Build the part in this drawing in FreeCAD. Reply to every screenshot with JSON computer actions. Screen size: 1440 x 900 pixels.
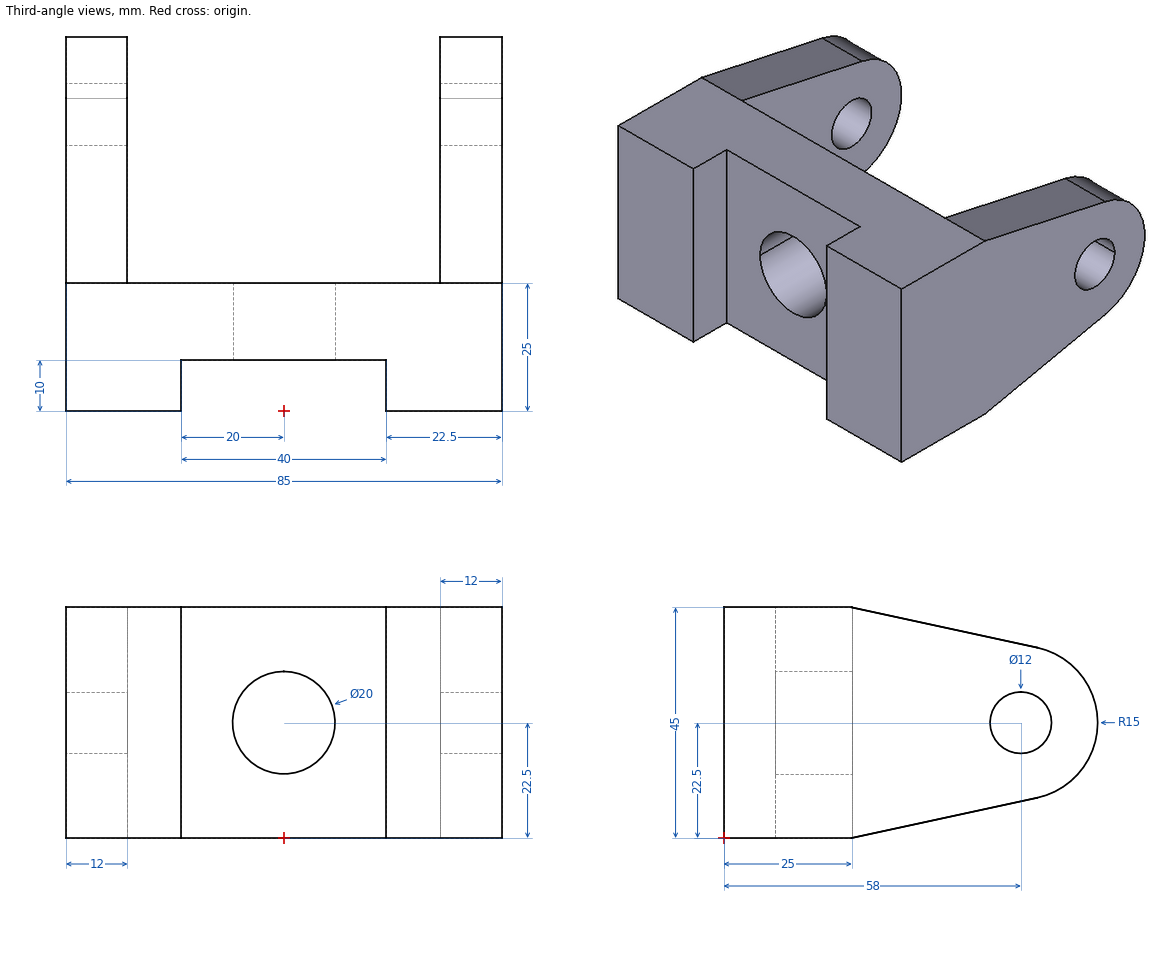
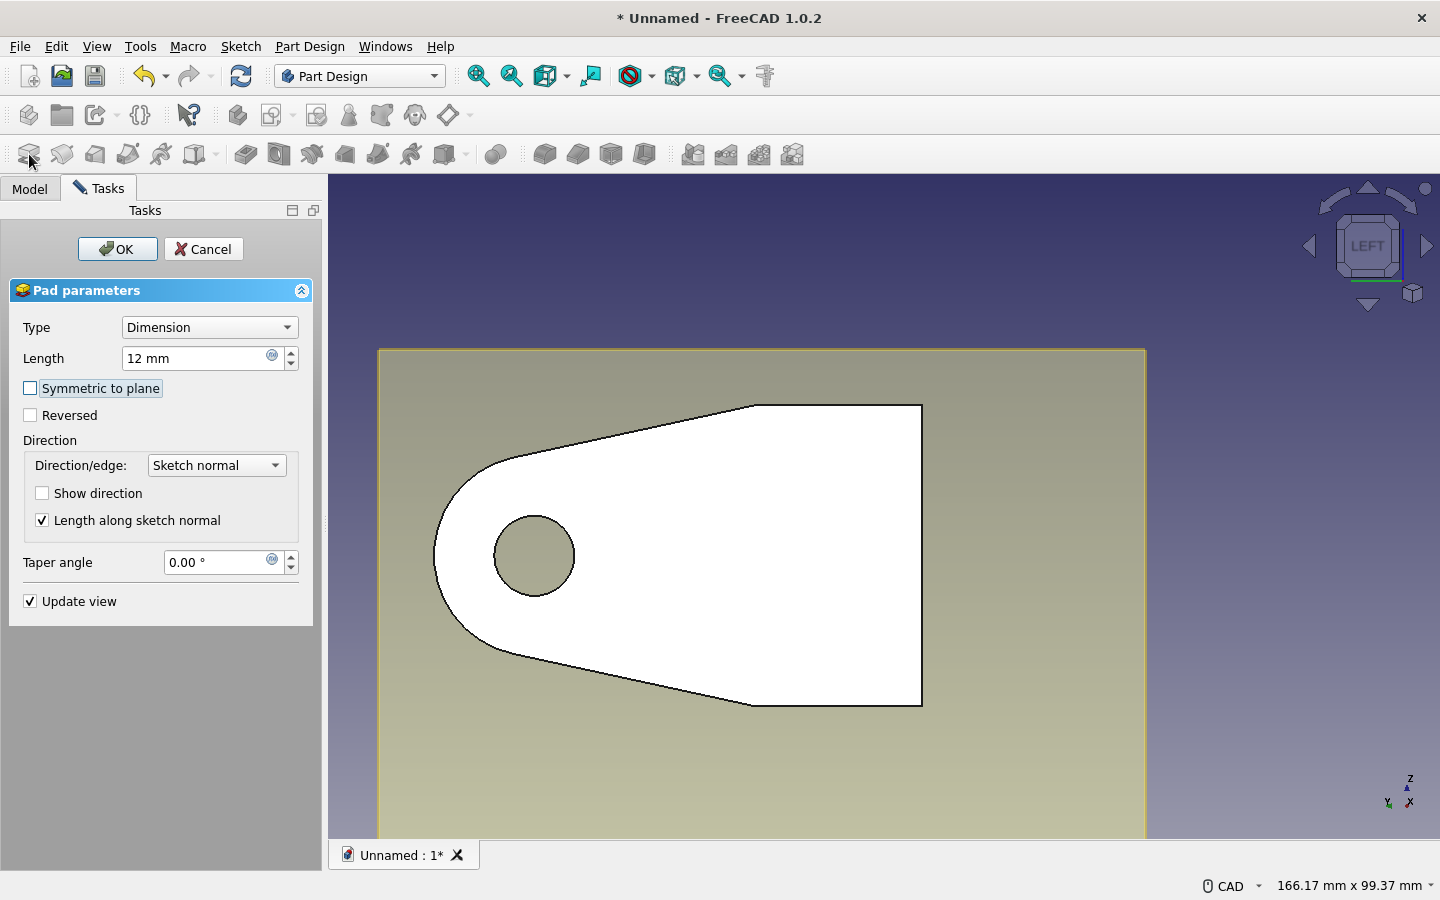
{"action": "left_click", "coordinate": [118, 249]}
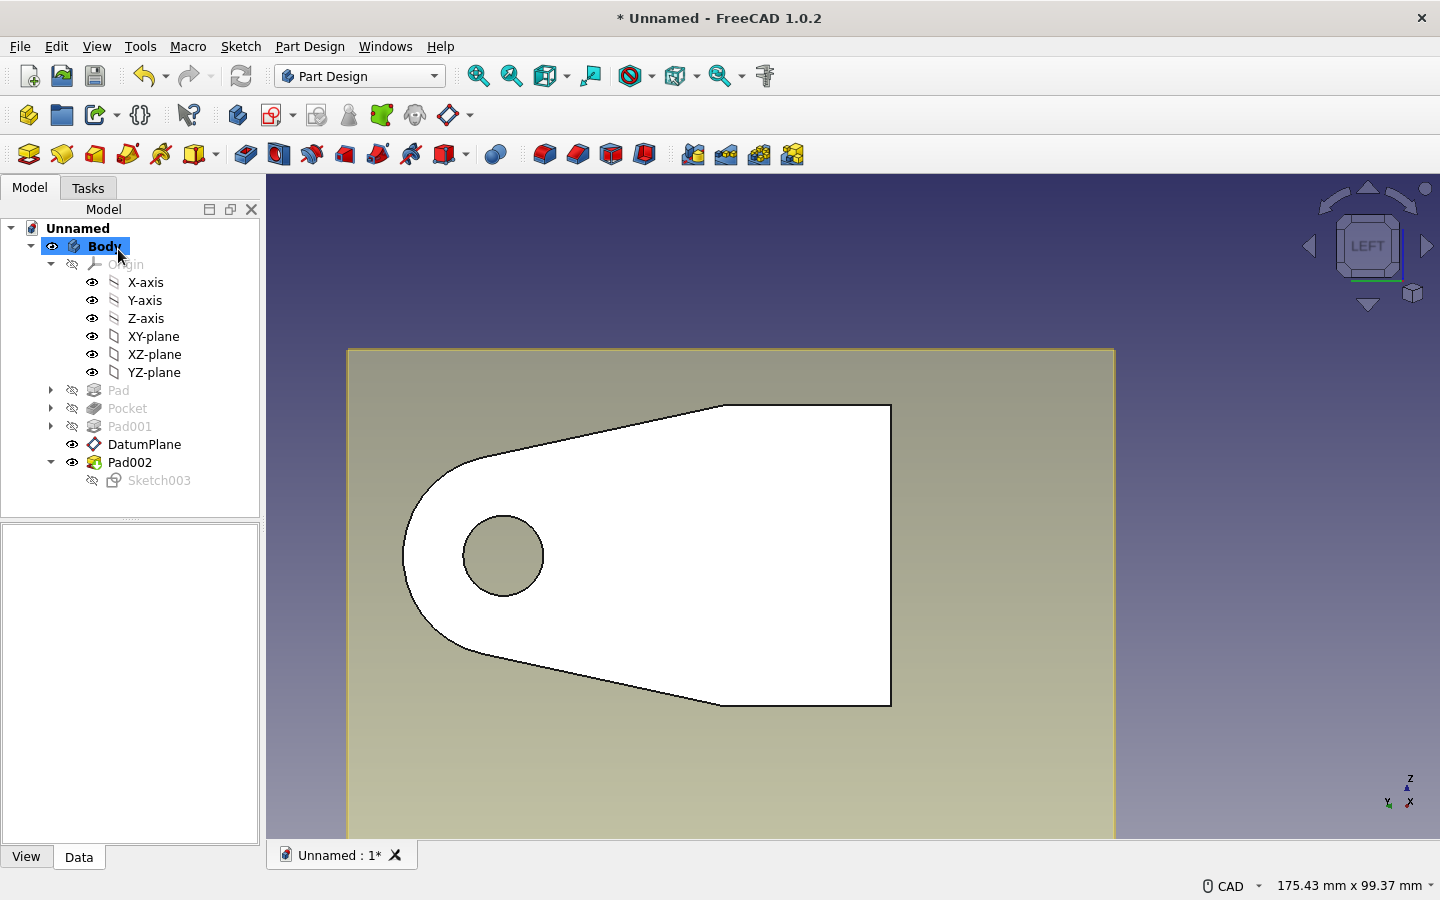
{"action": "left_click", "coordinate": [117, 444]}
{"action": "key", "text": "space"}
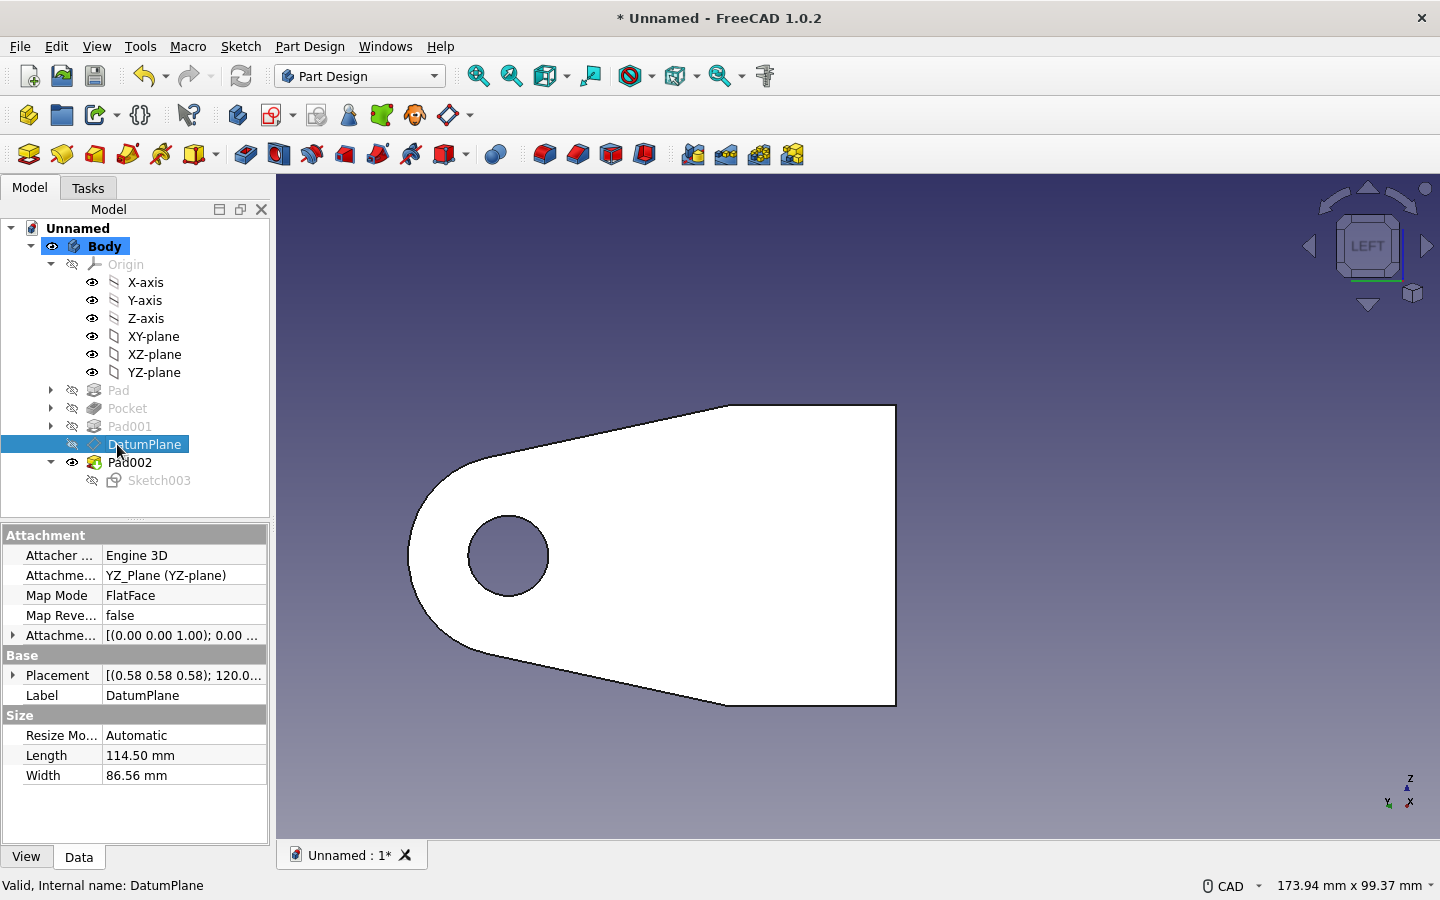
{"action": "key", "text": "0"}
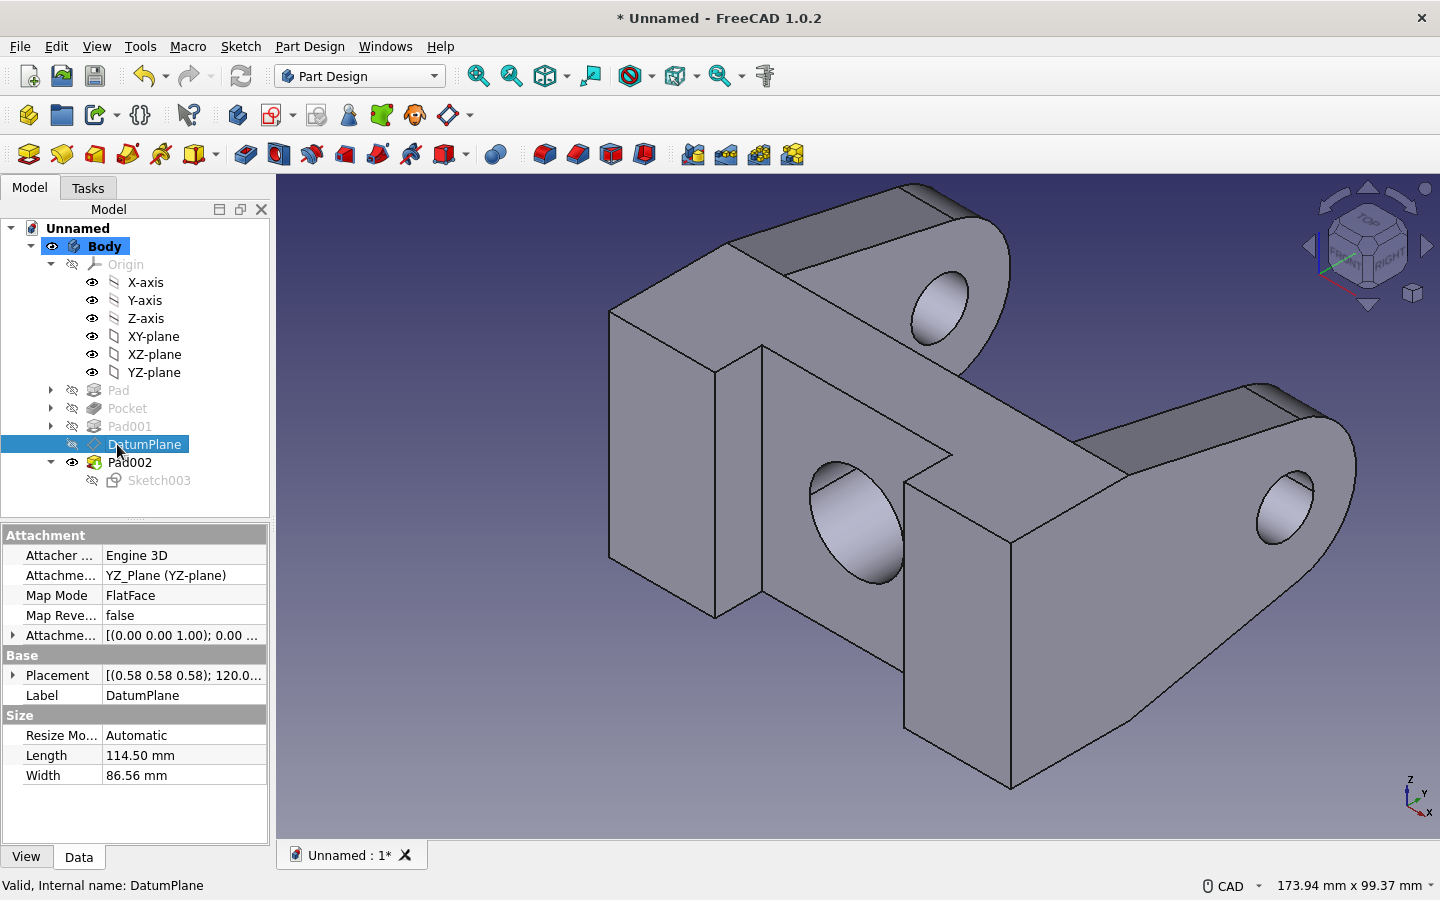
{"action": "left_click", "coordinate": [479, 76]}